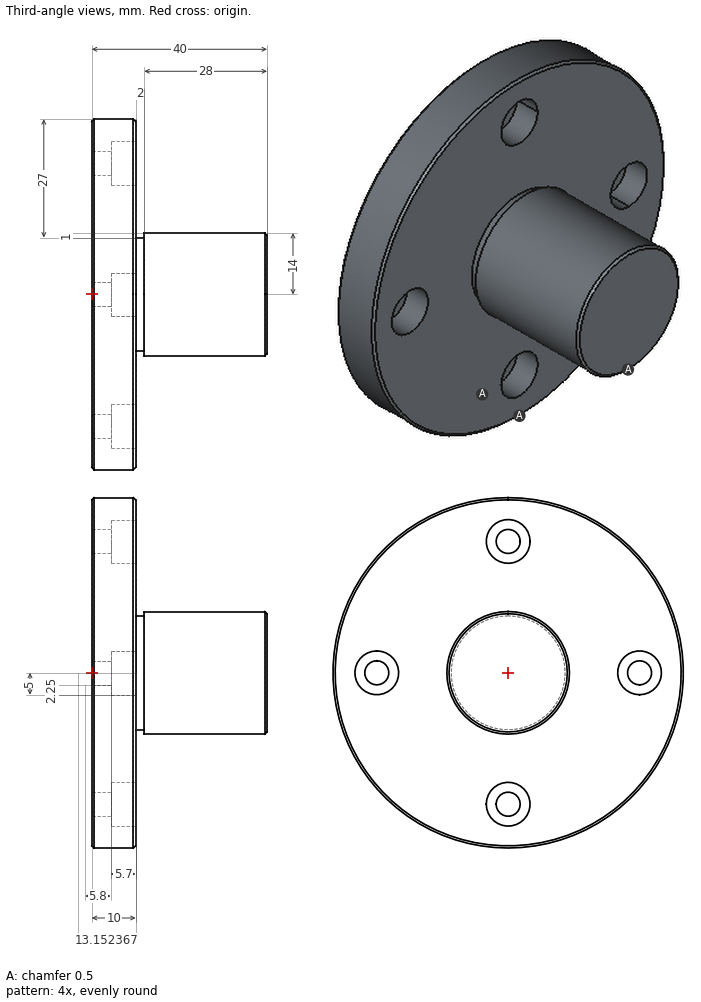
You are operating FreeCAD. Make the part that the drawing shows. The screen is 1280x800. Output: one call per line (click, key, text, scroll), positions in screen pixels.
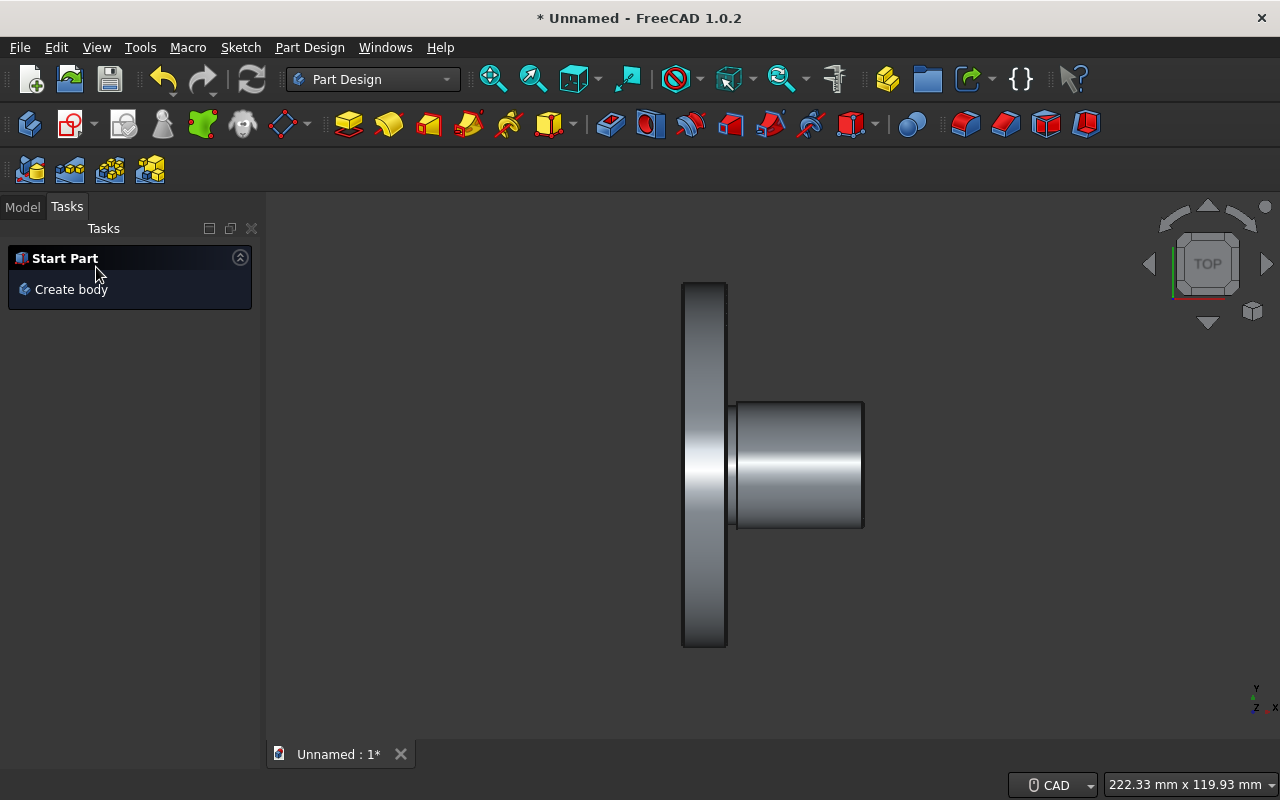
click(23, 206)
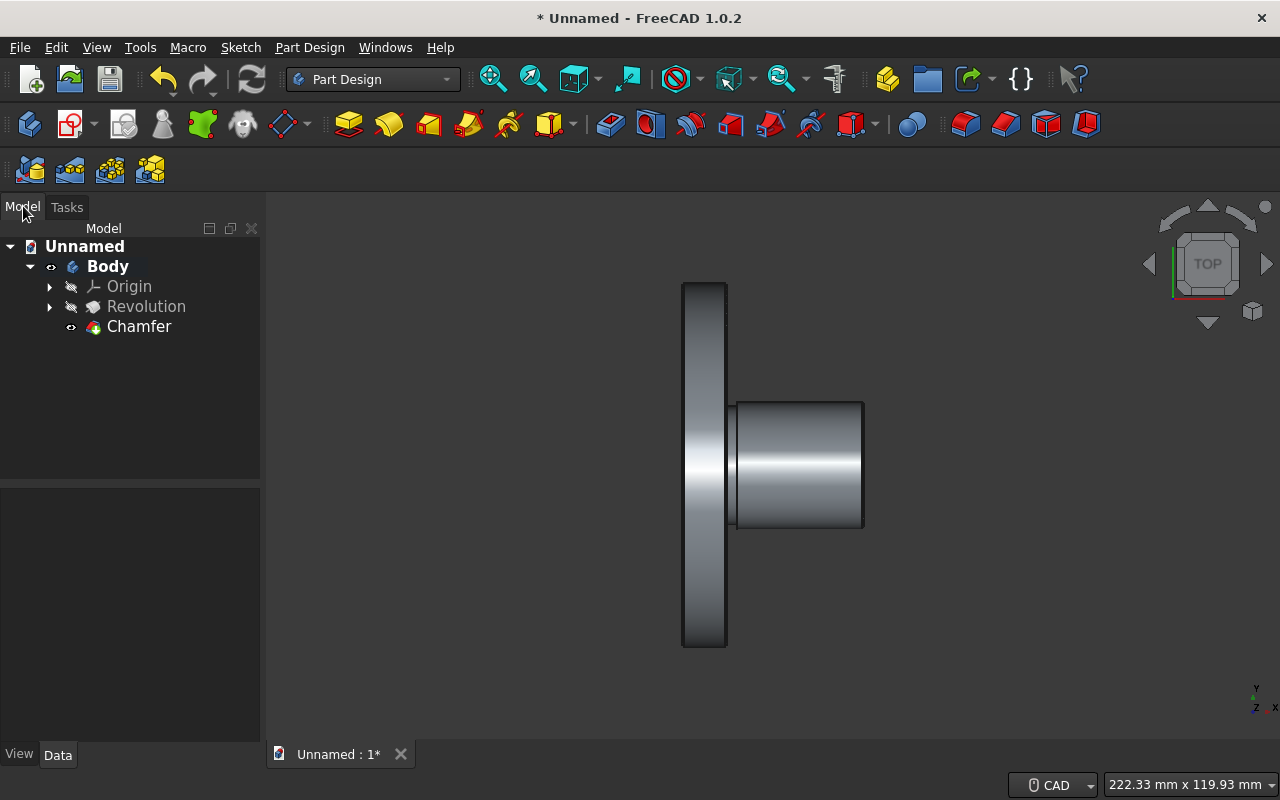
click(50, 287)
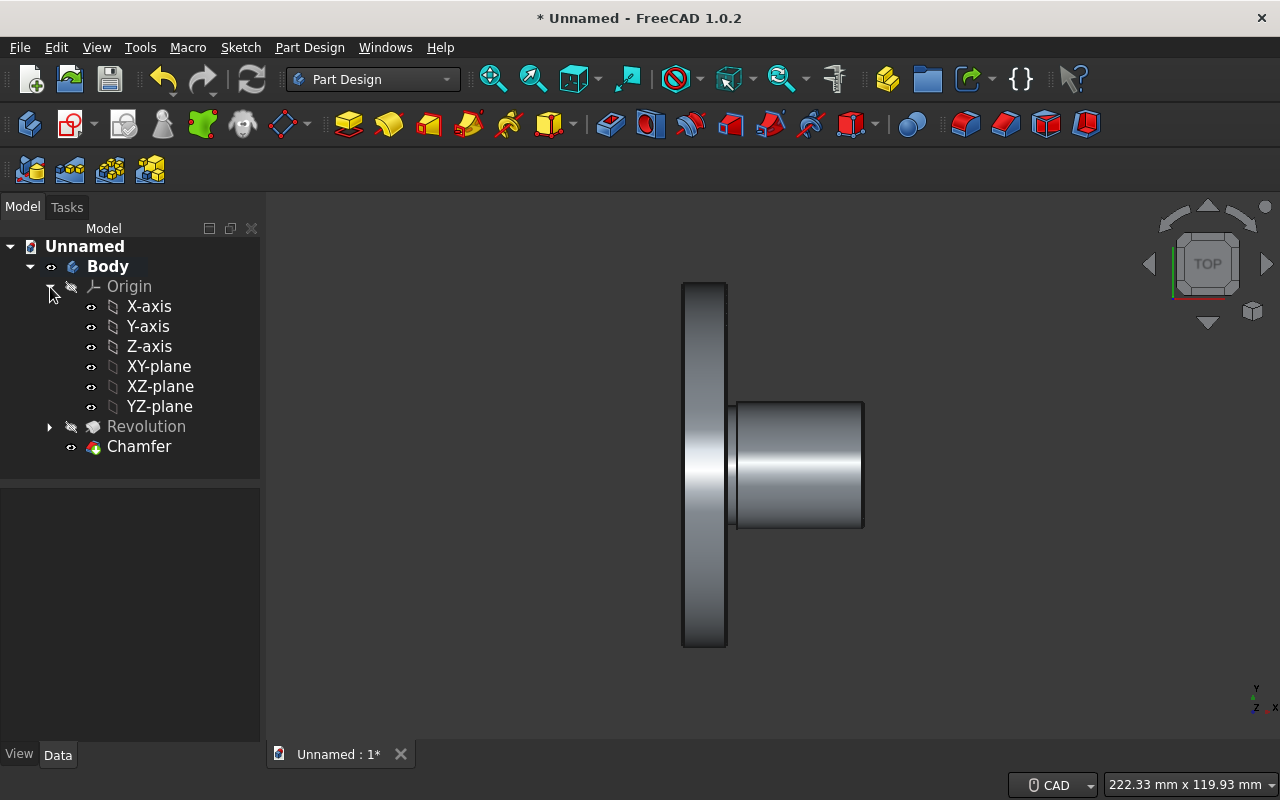
click(136, 387)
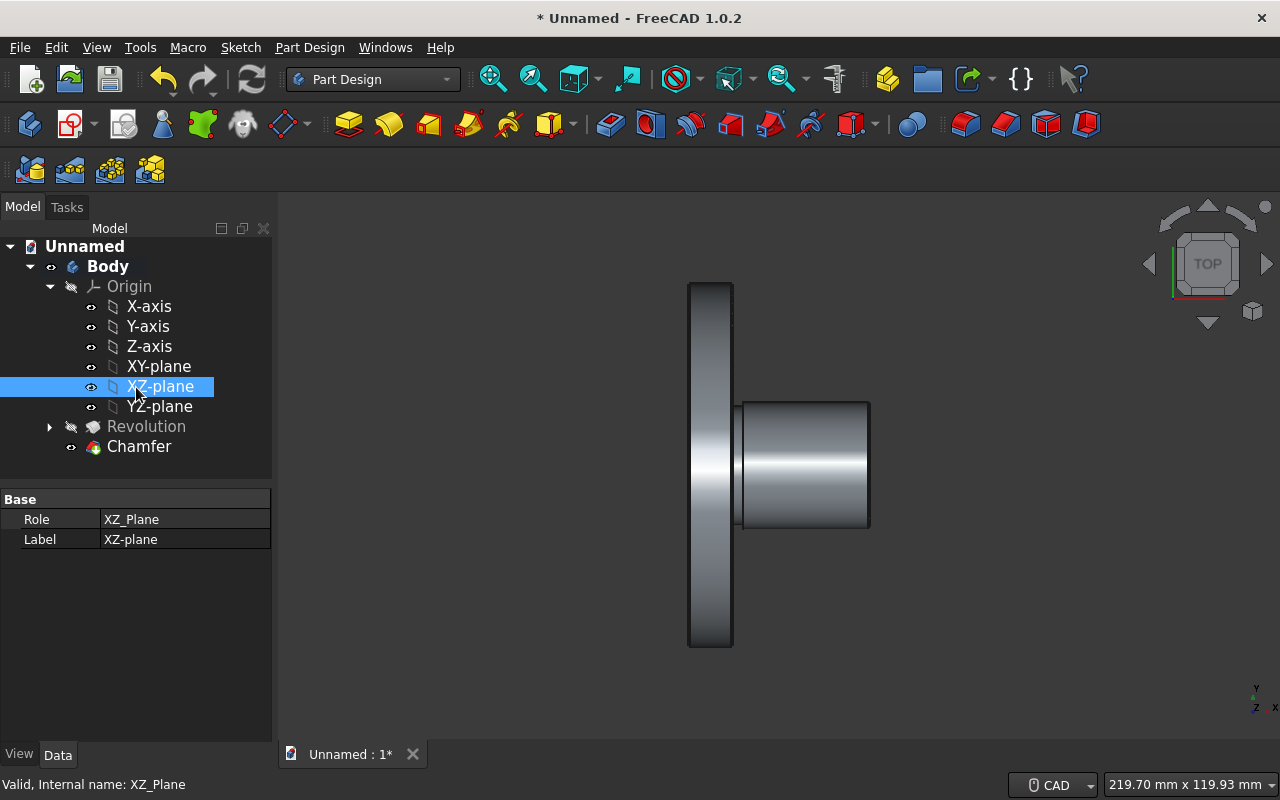
click(284, 124)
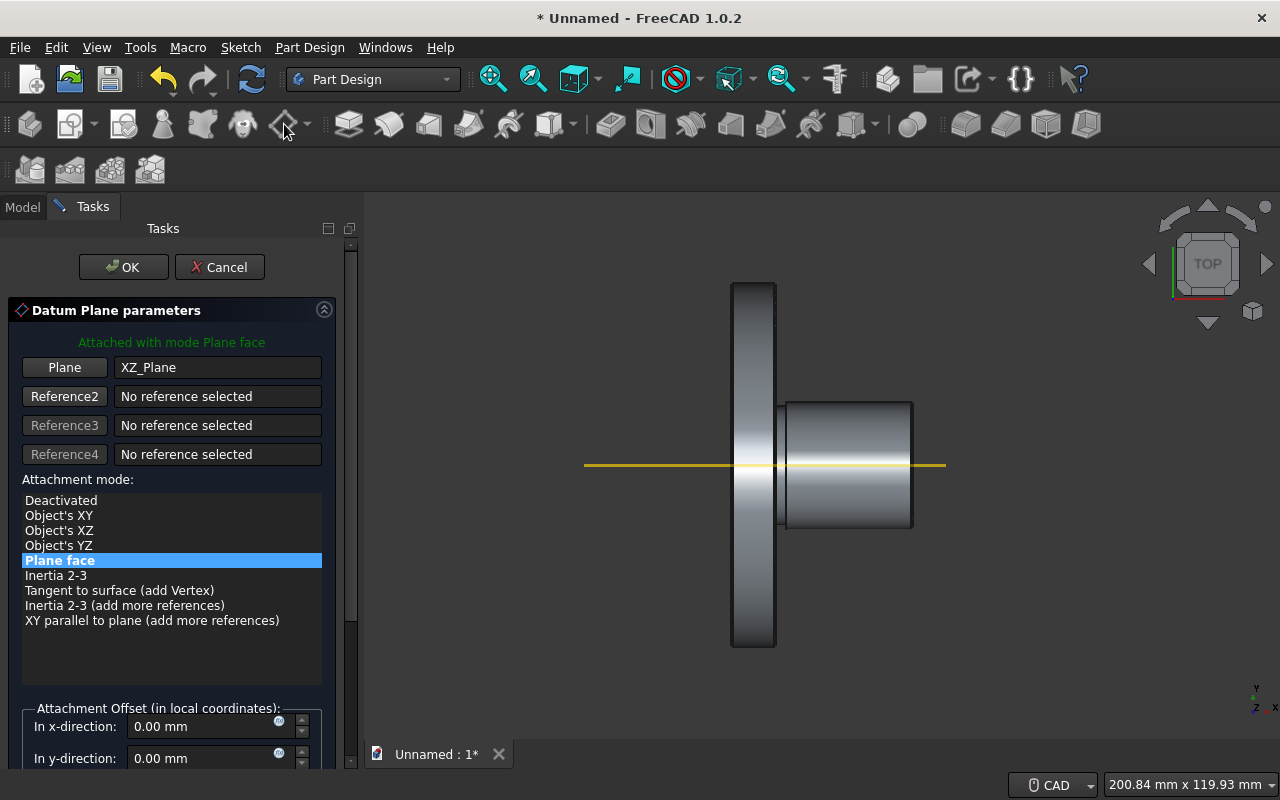
scroll(351, 503, down, 2)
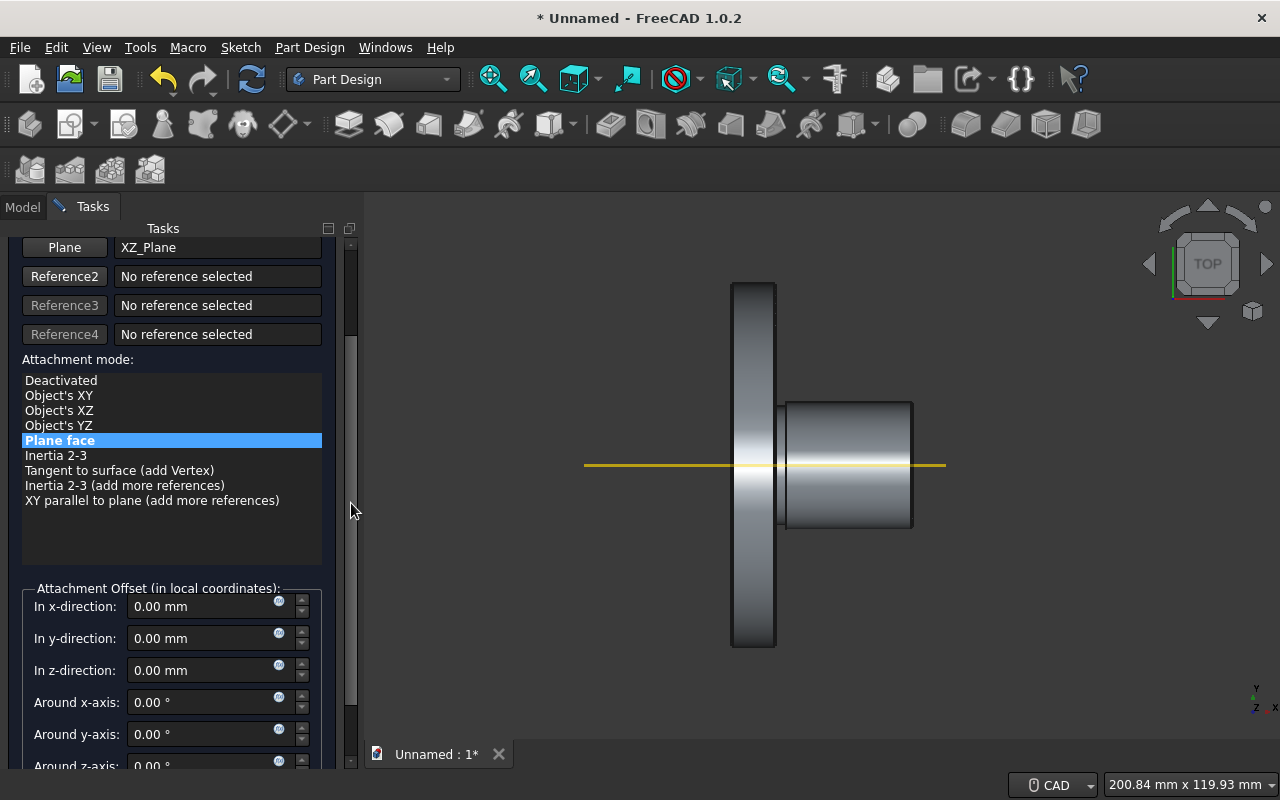
triple_click(210, 670)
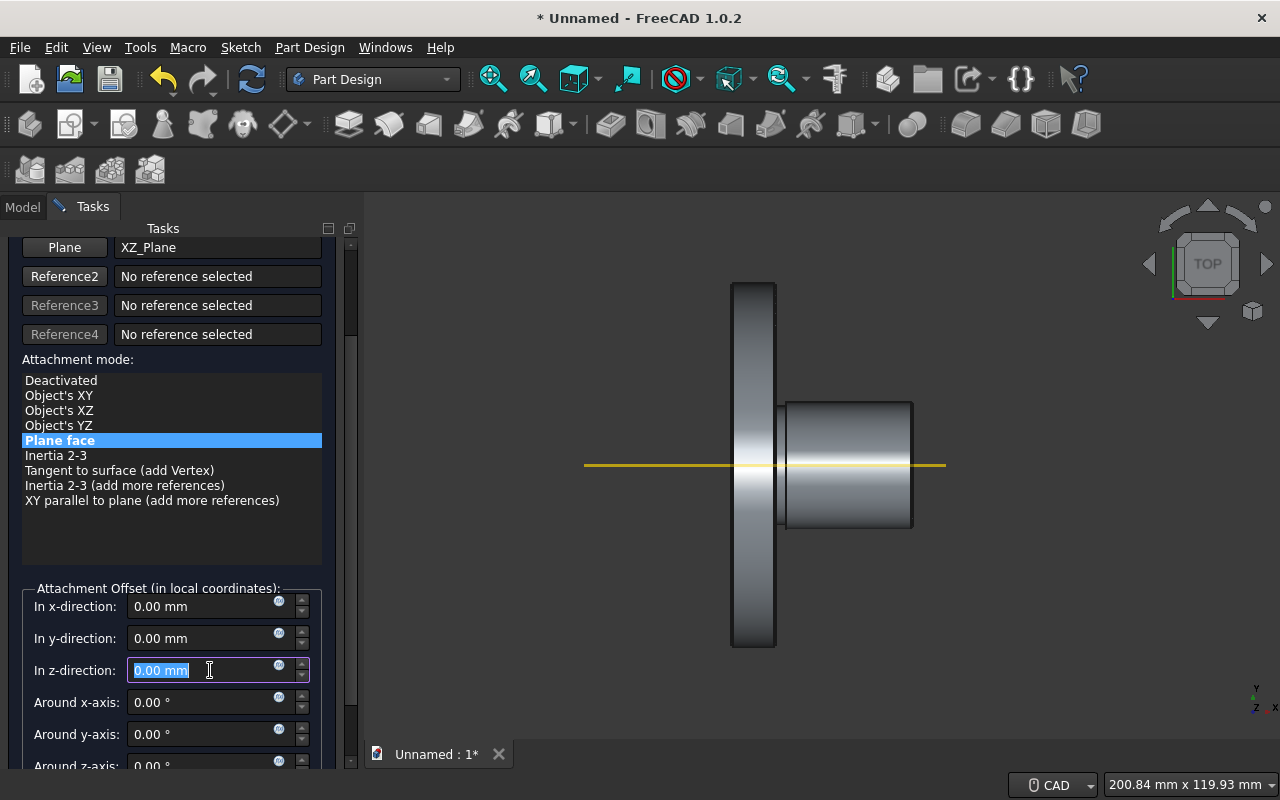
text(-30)
key(Tab)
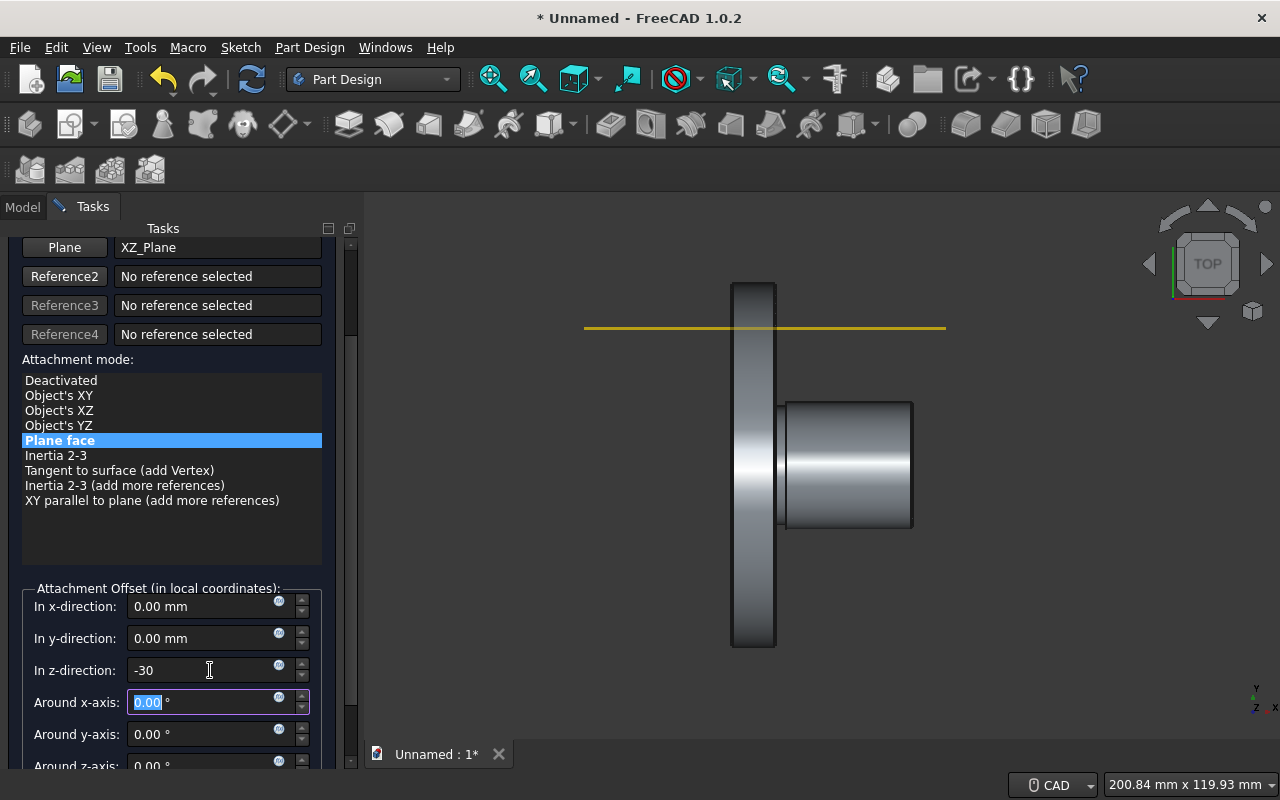
scroll(351, 503, up, 3)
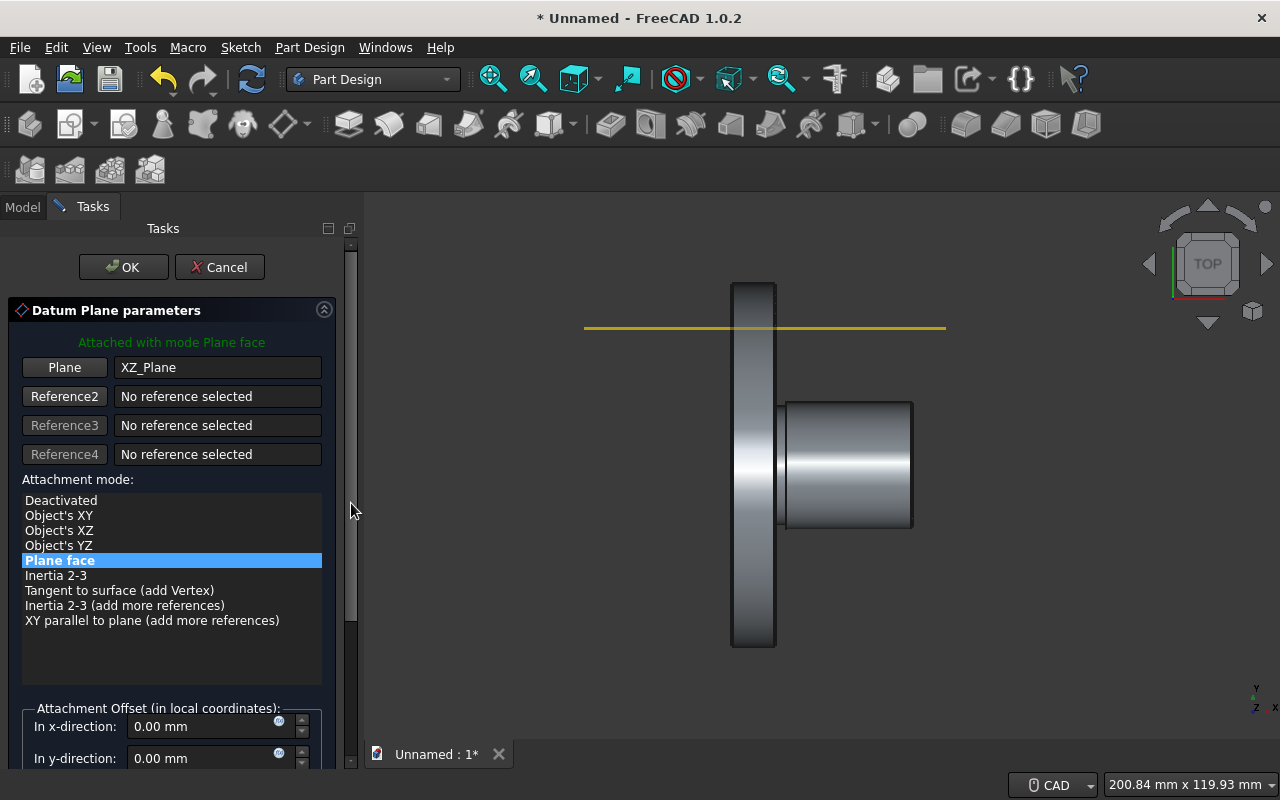
click(124, 267)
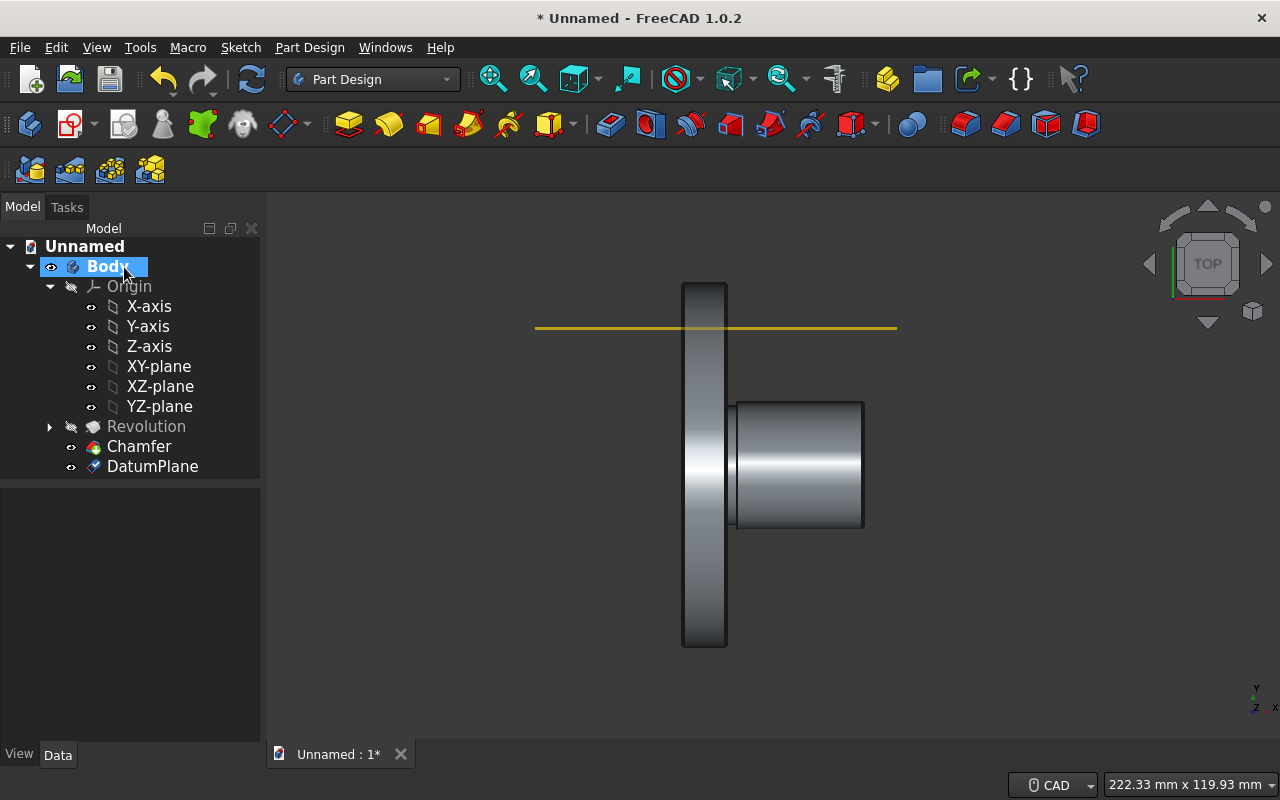
click(116, 467)